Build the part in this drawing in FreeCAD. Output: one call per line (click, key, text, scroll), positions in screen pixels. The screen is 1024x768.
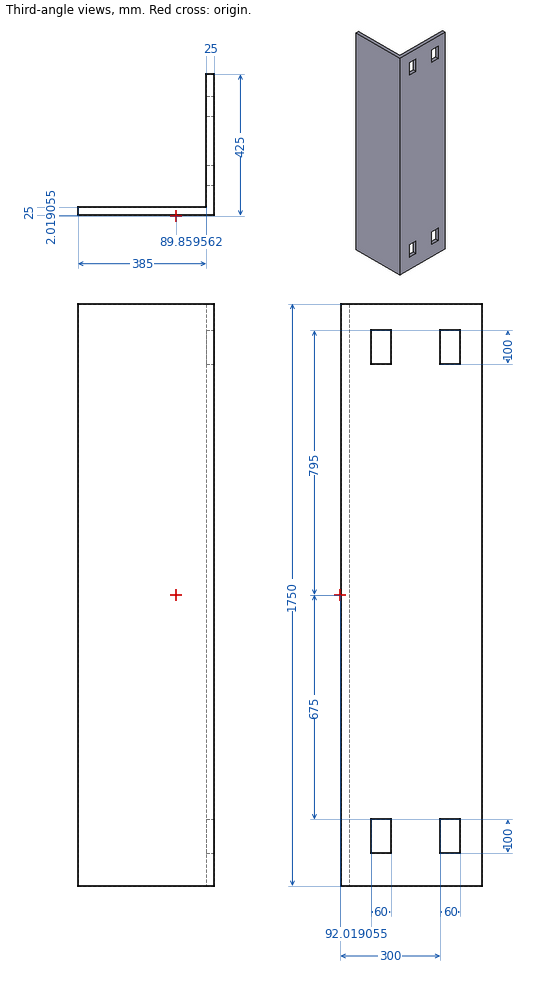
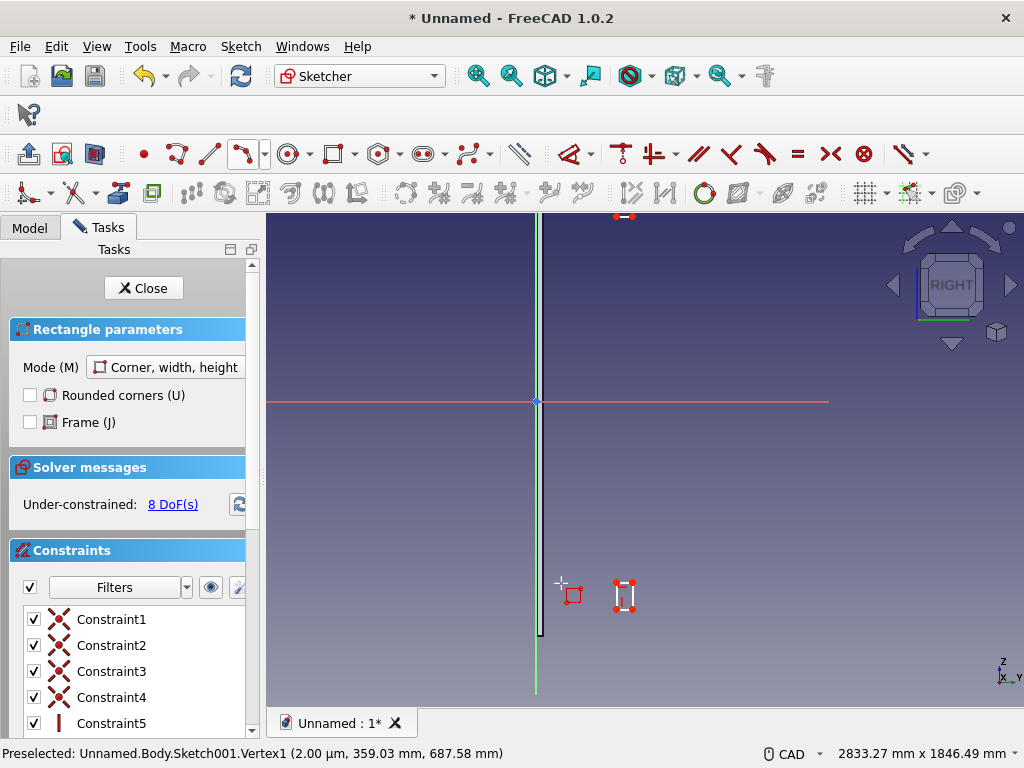
click(561, 582)
click(577, 609)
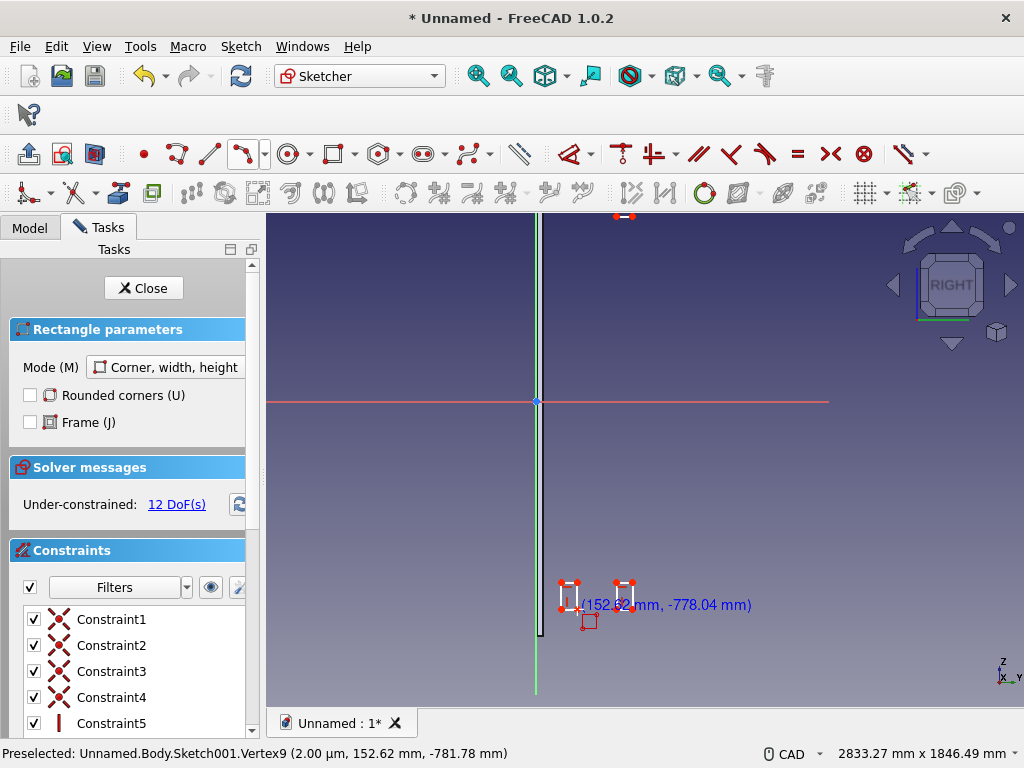
scroll(561, 584, down, 2)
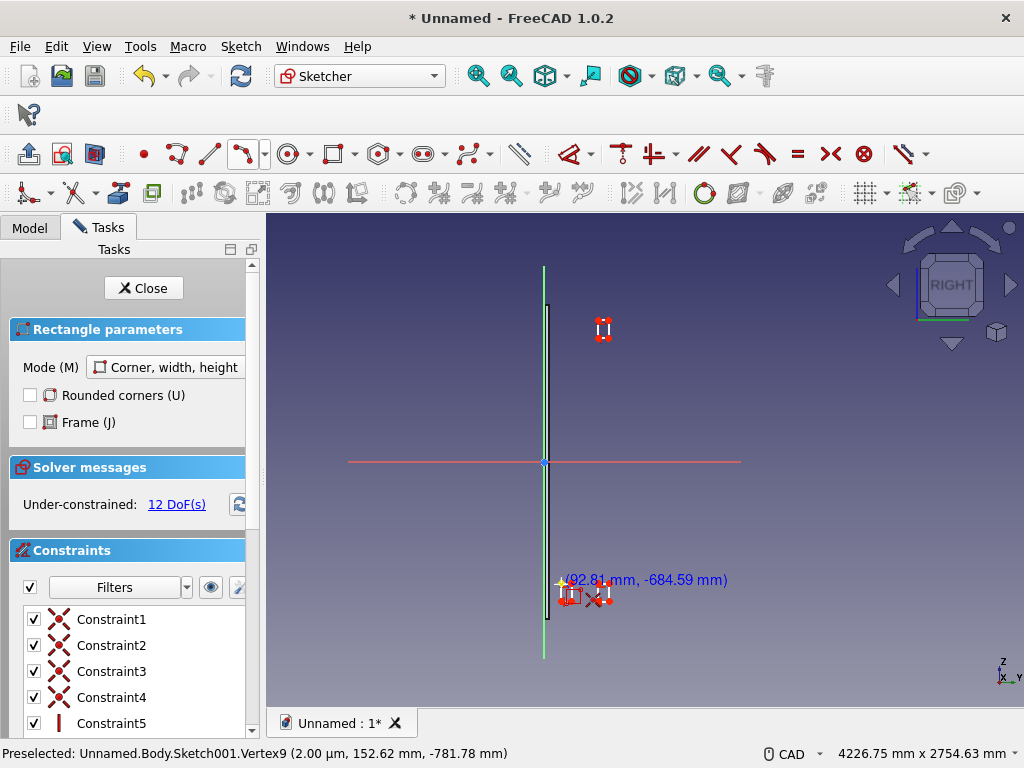
scroll(561, 320, up, 2)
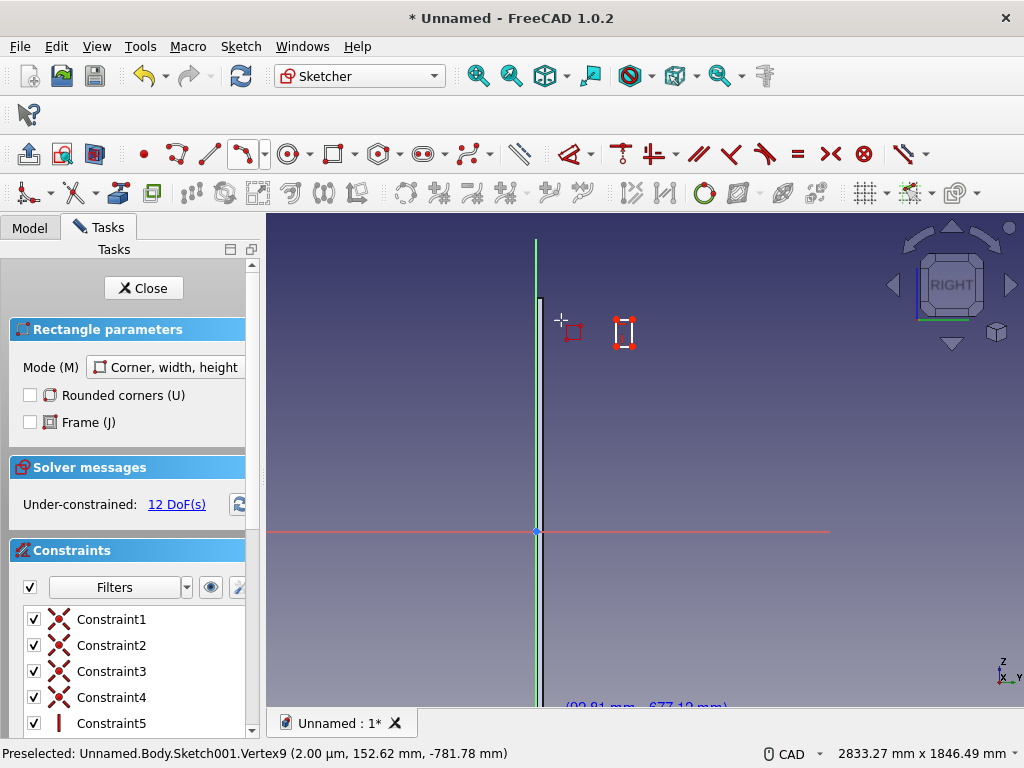
click(561, 319)
click(577, 346)
key(Escape)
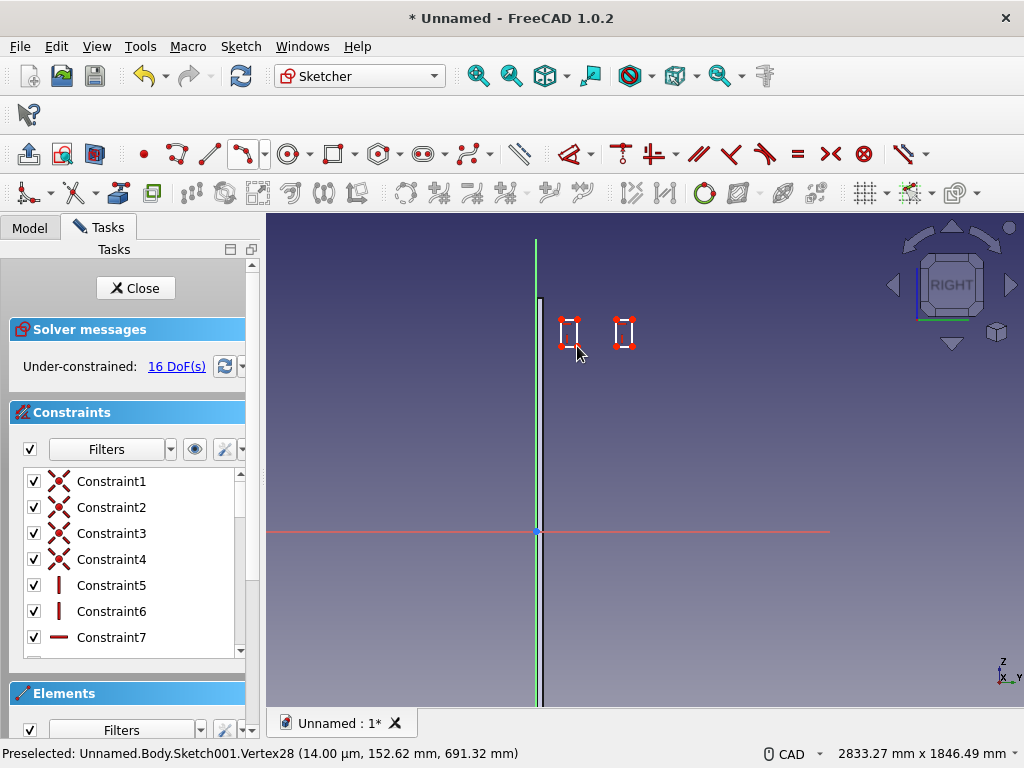
click(568, 154)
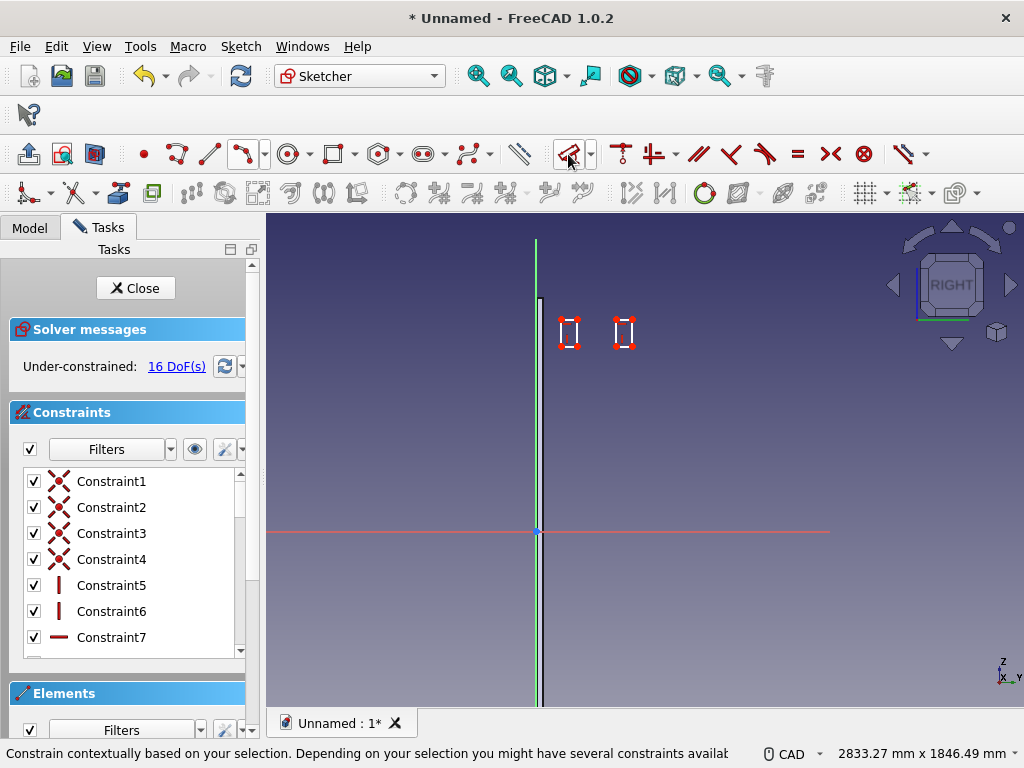
scroll(561, 319, down, 2)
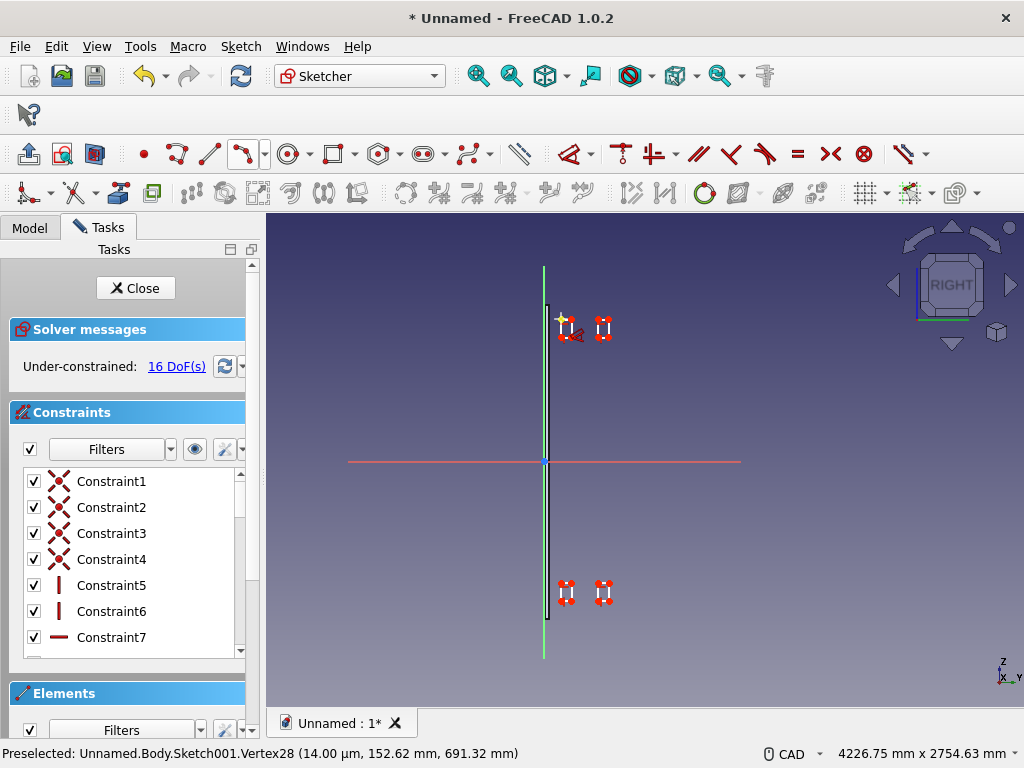
scroll(604, 601, up, 7)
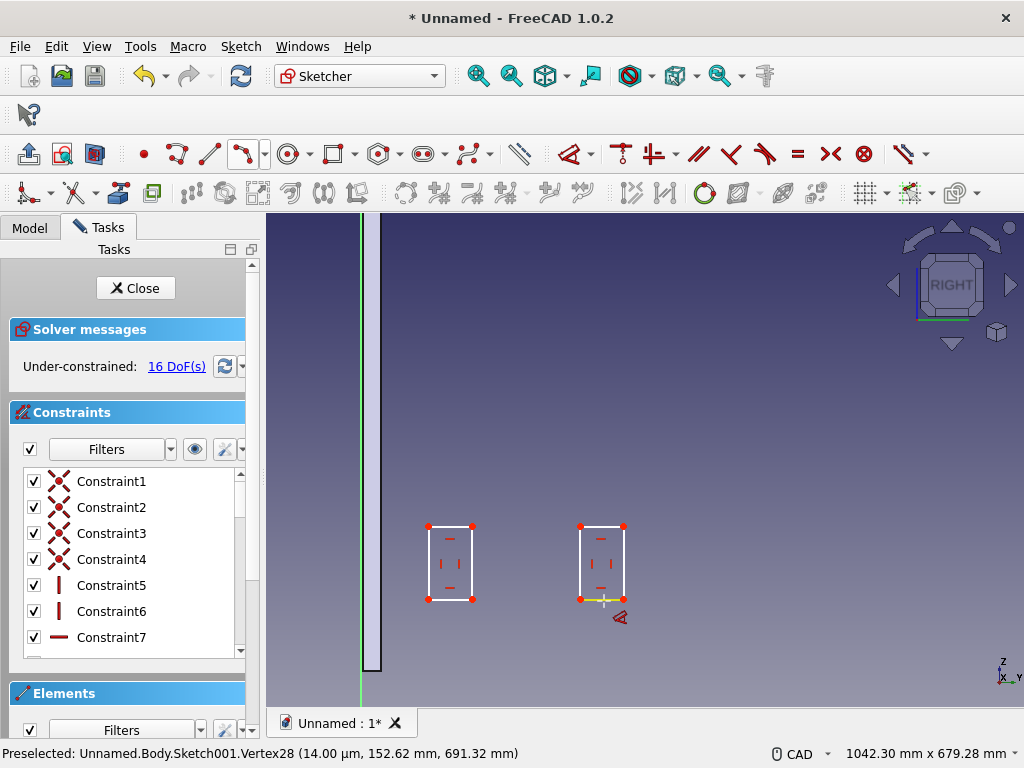
click(602, 600)
click(602, 634)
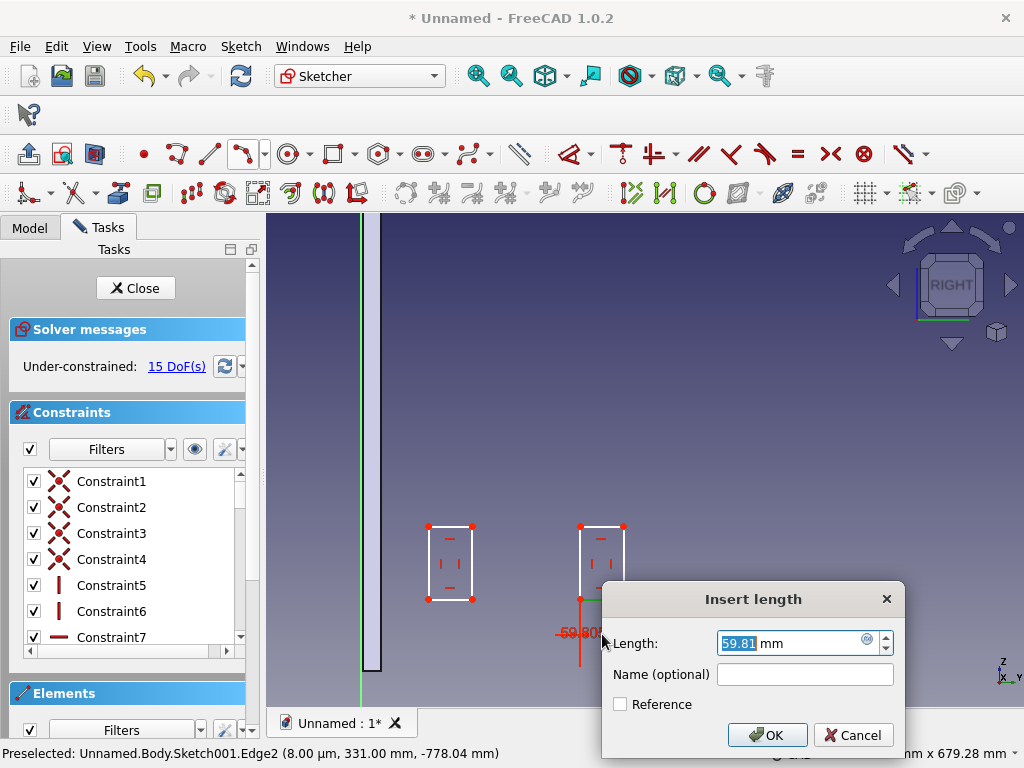
text(60)
key(Return)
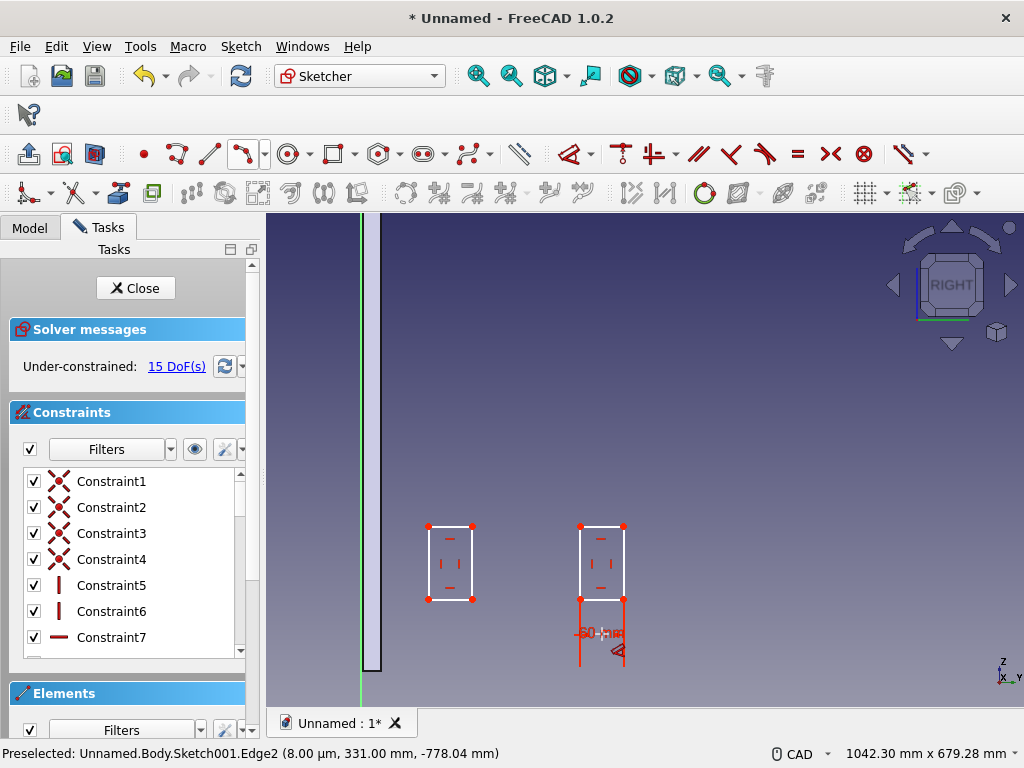
scroll(604, 602, down, 7)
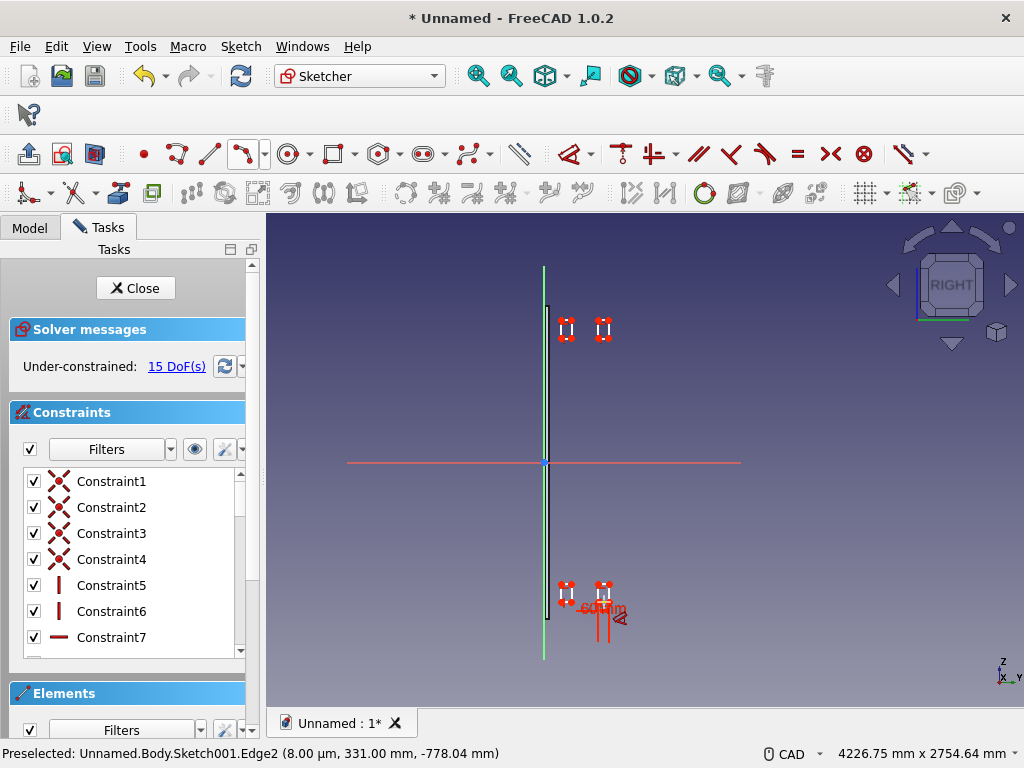
scroll(601, 339, up, 8)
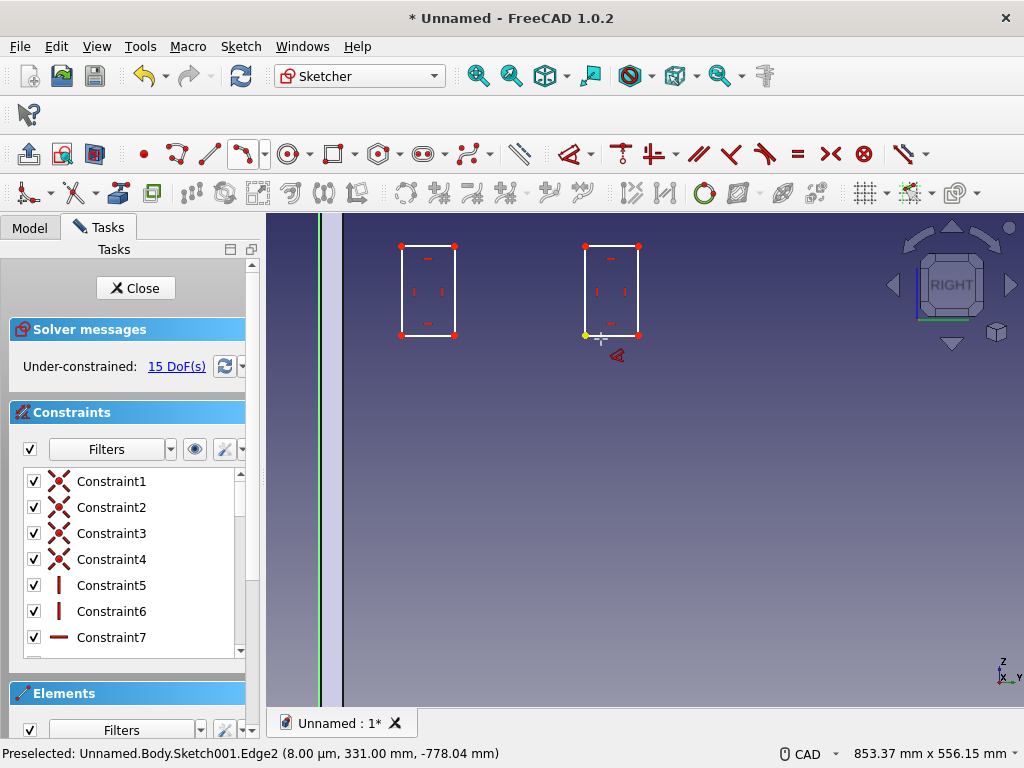
click(601, 336)
click(612, 302)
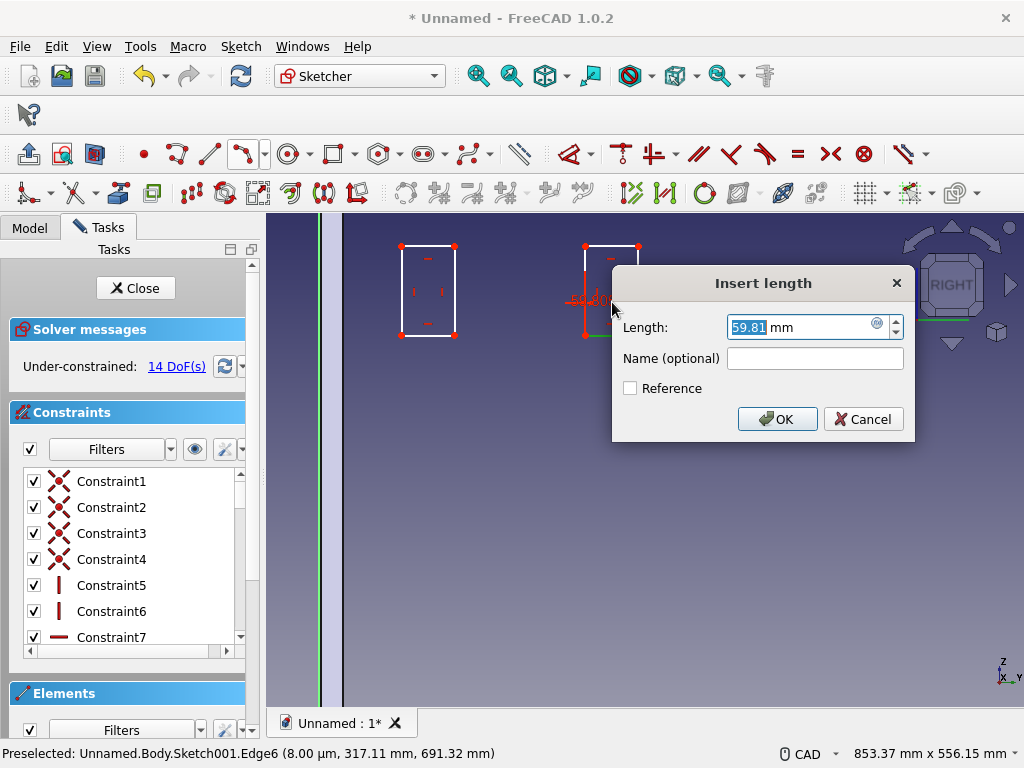
text(60)
key(Return)